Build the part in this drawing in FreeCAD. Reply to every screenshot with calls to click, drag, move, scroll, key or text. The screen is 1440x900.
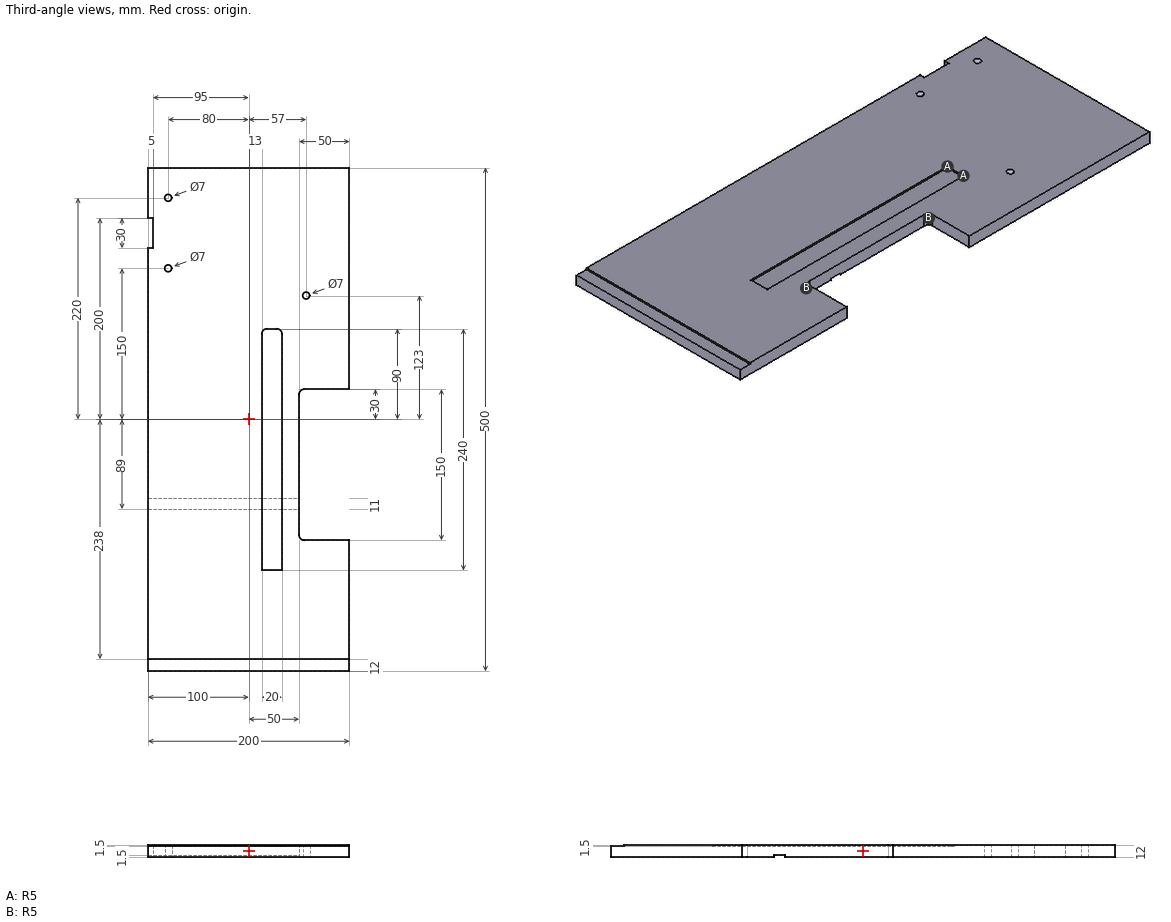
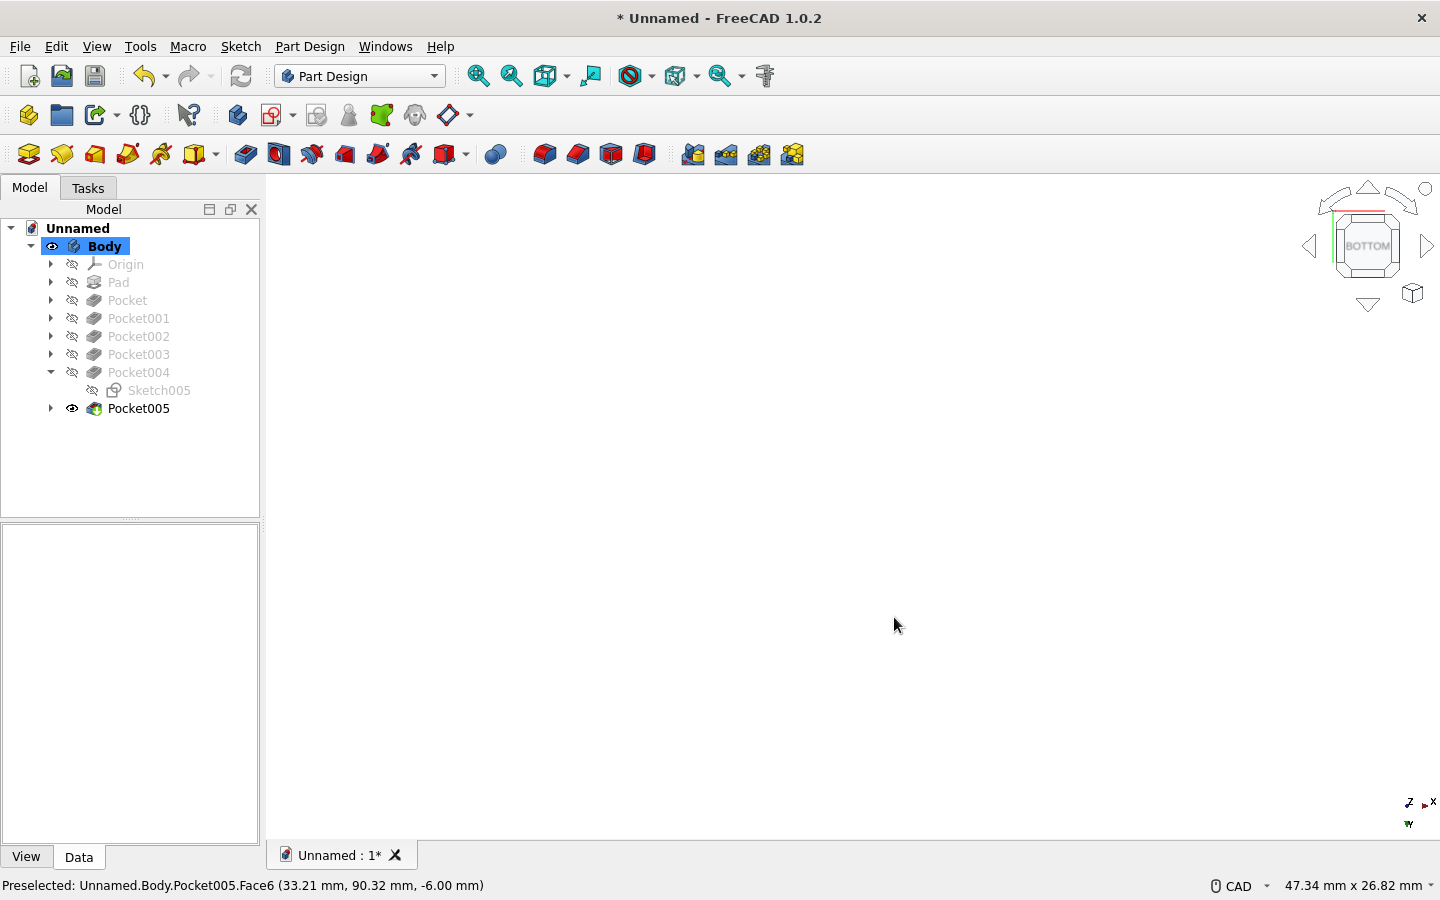
click(479, 76)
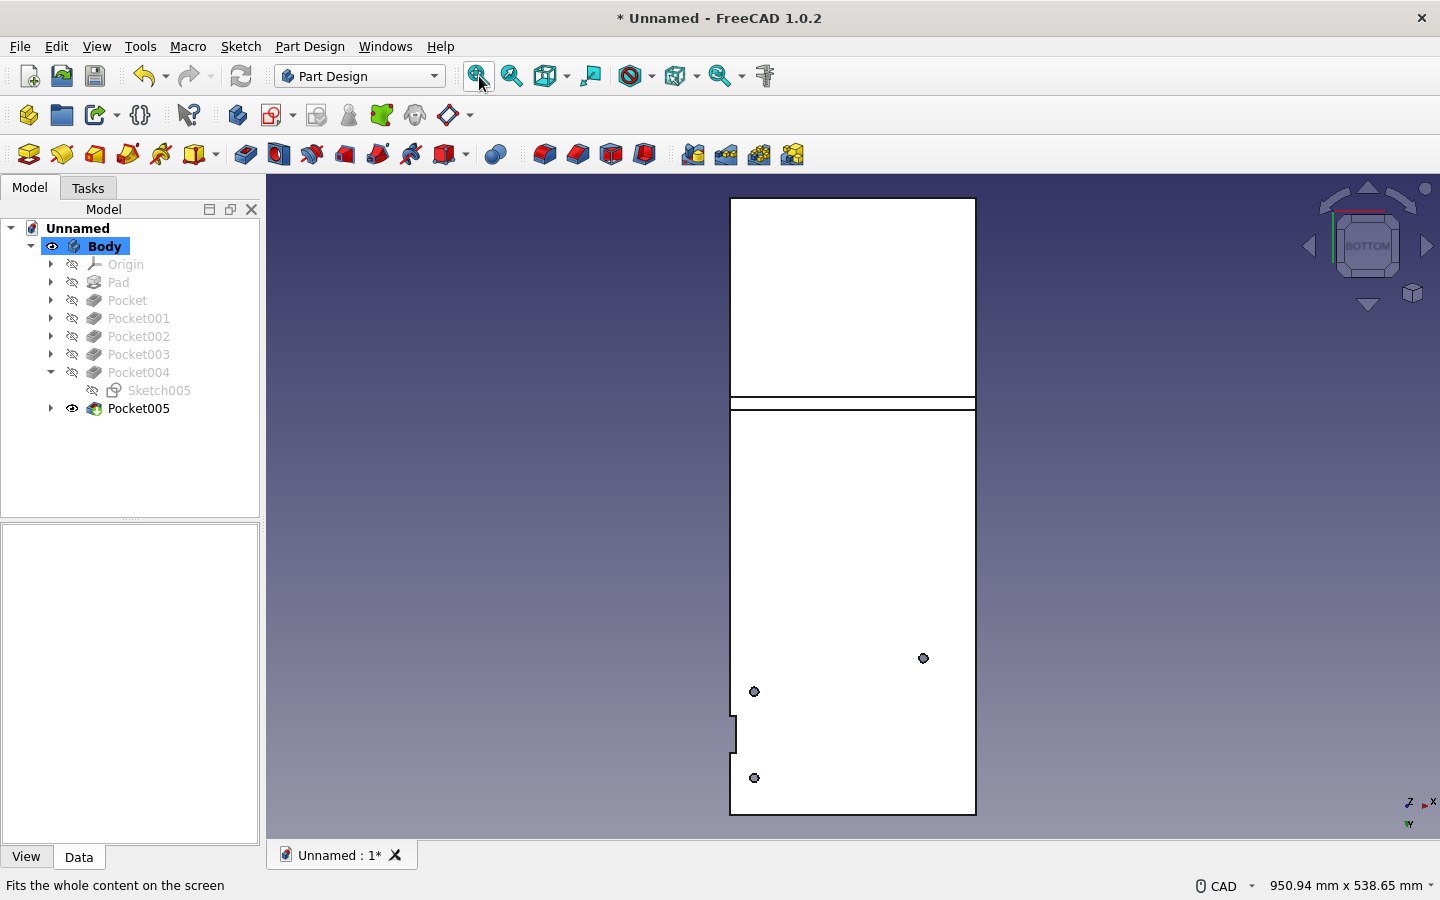
key(4)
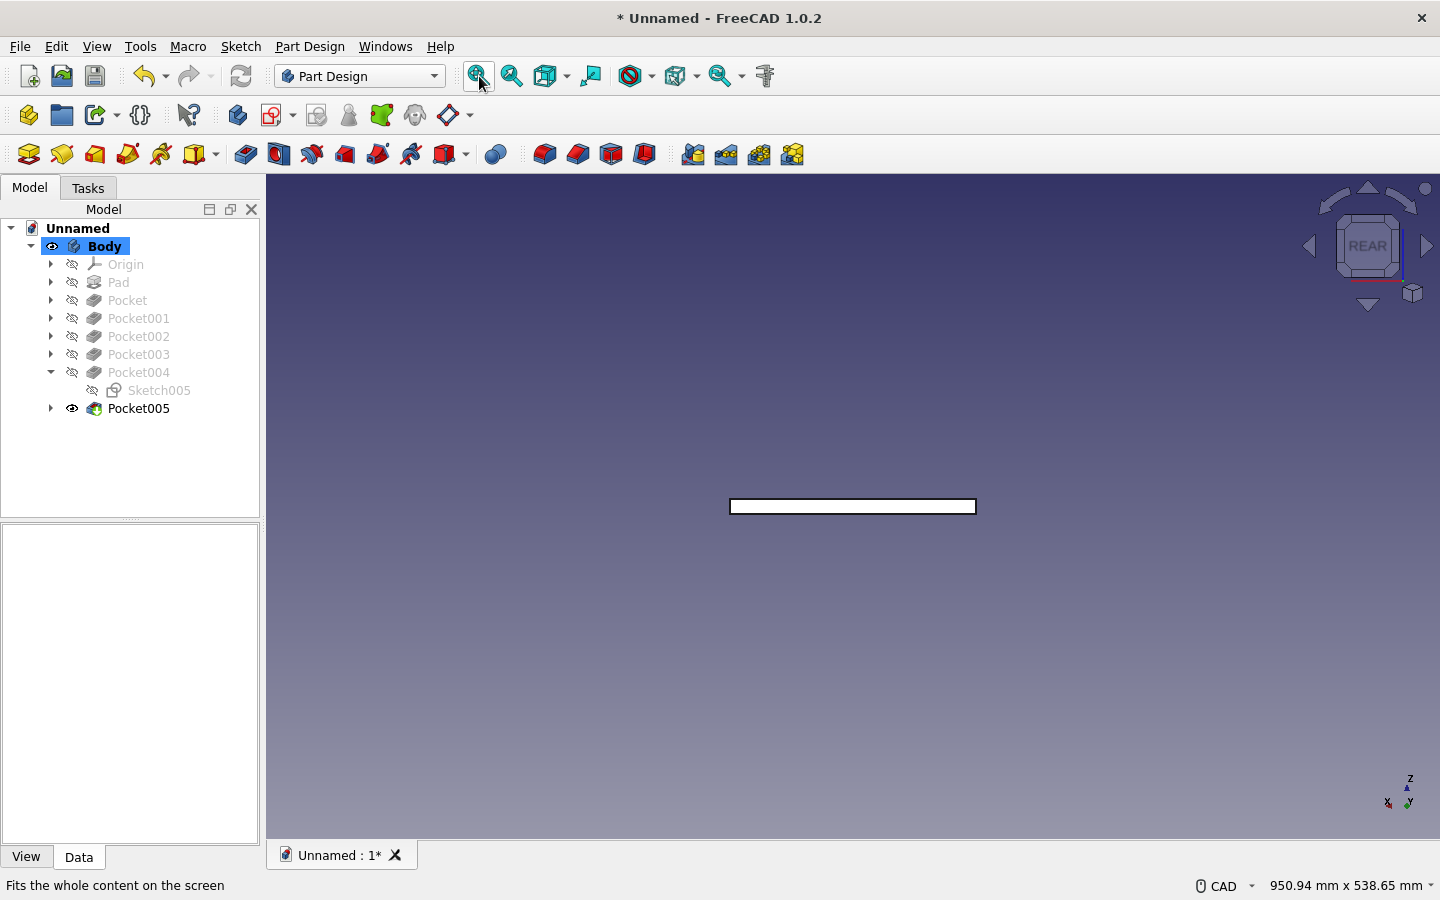
click(479, 76)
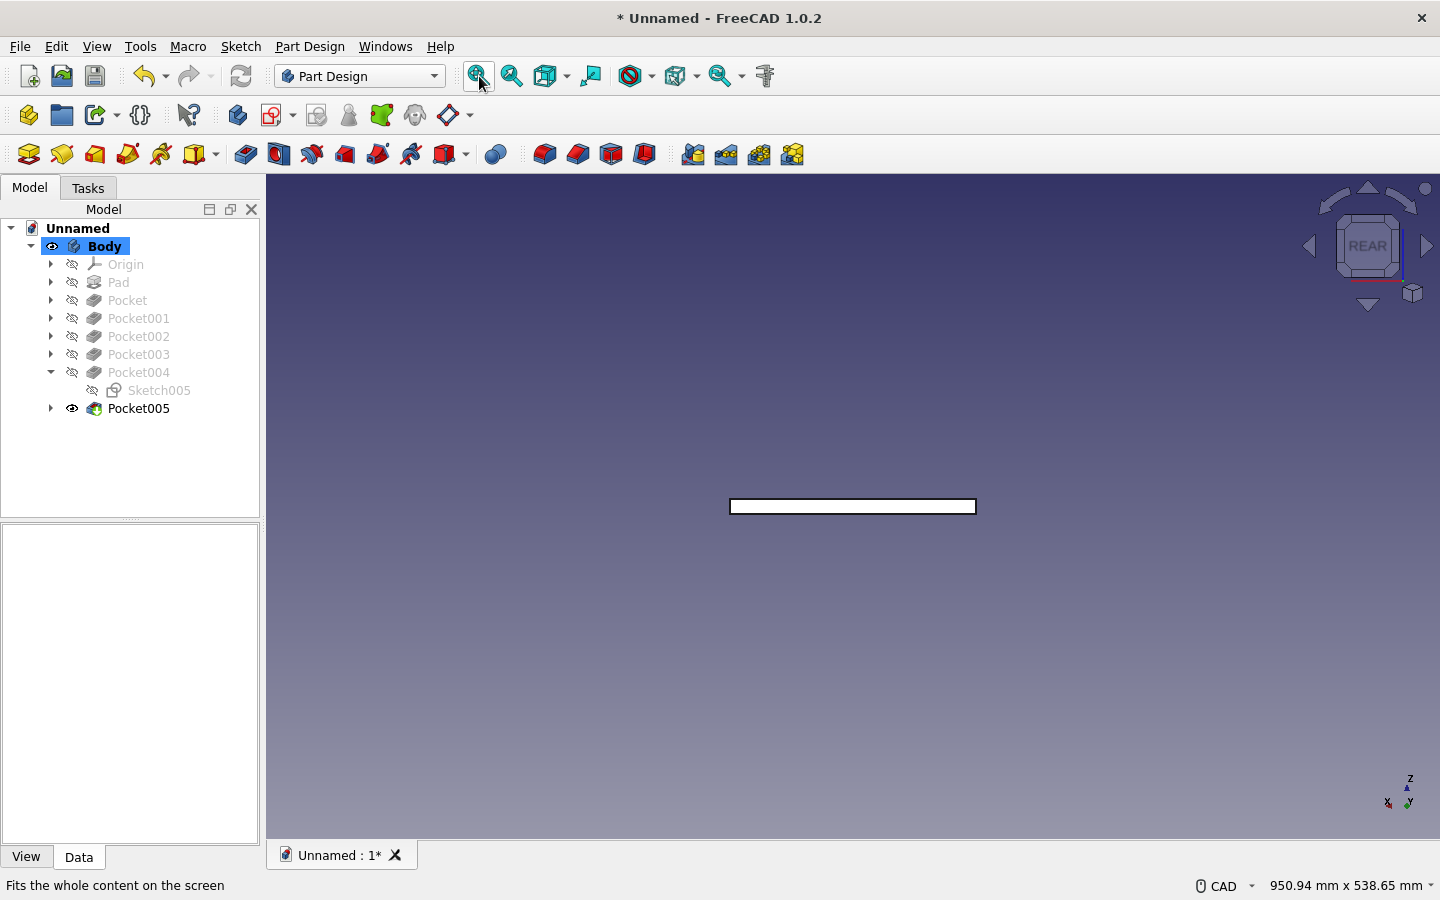
scroll(812, 499, up, 15)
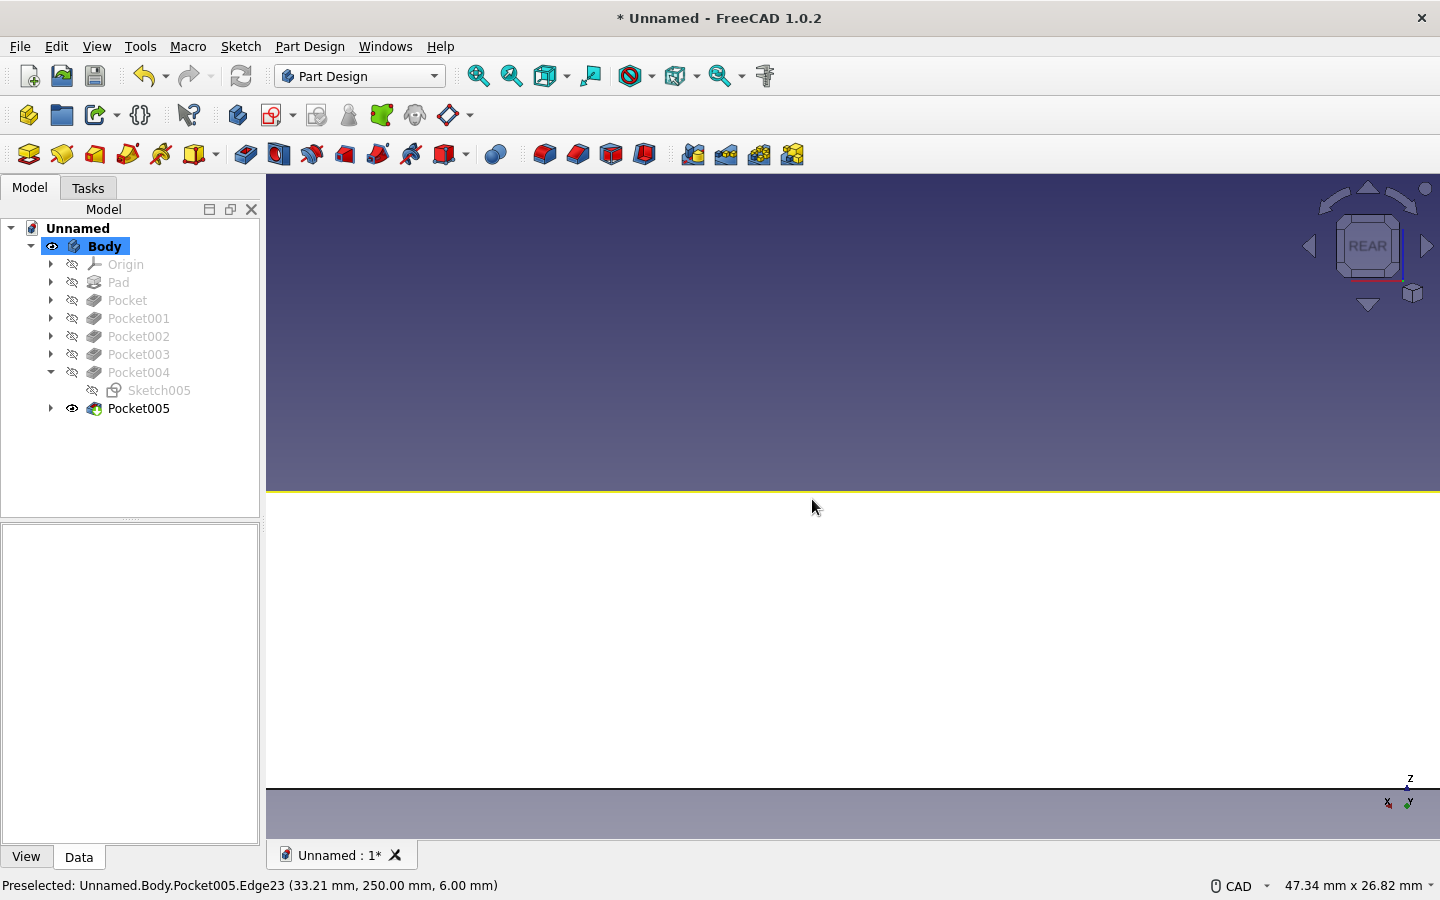
click(479, 76)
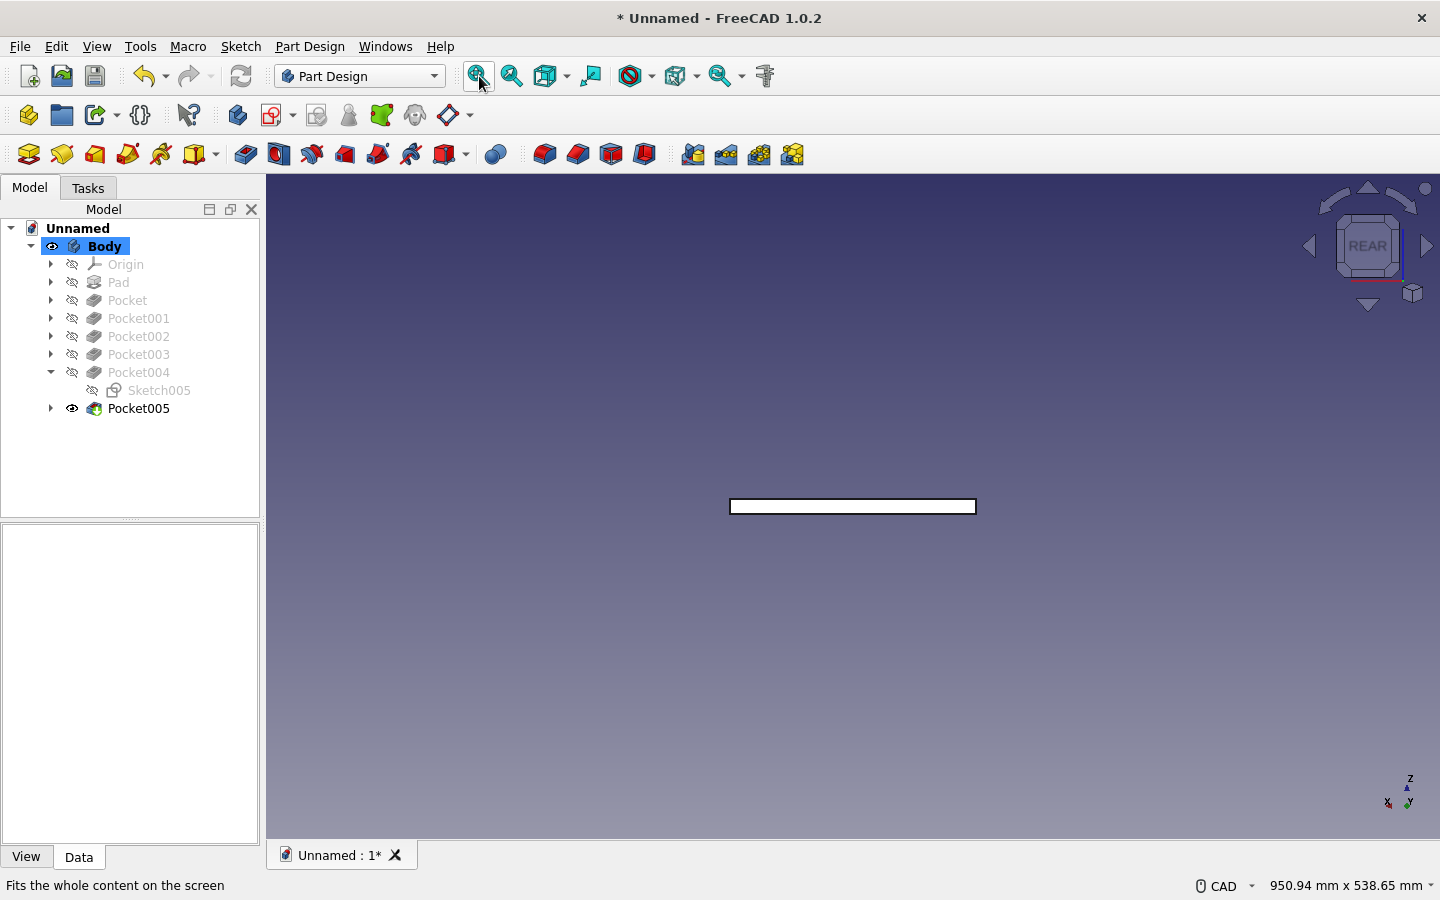
key(6)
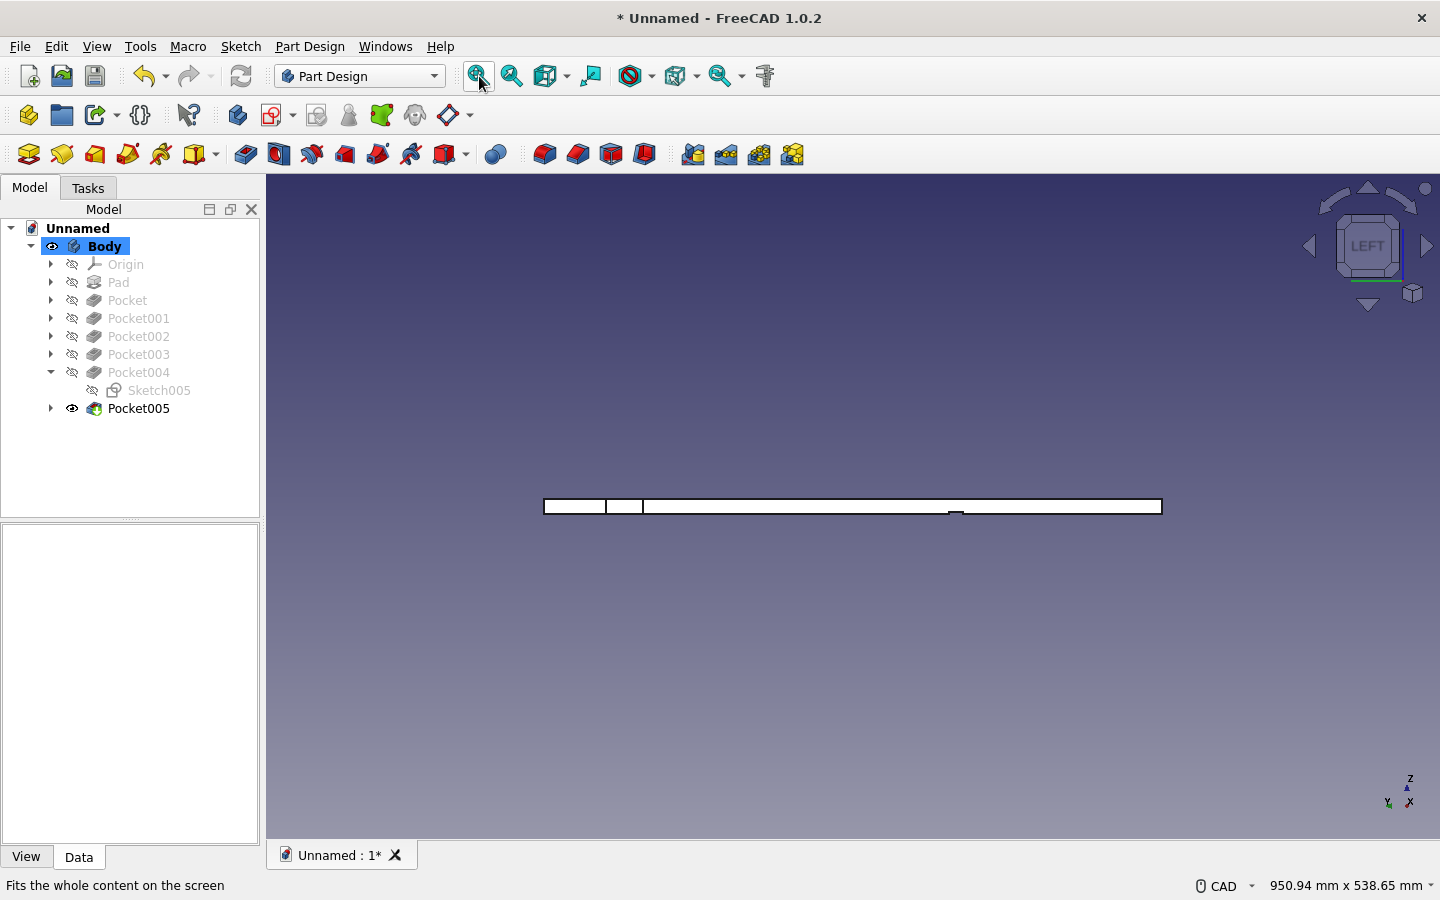
scroll(742, 499, up, 15)